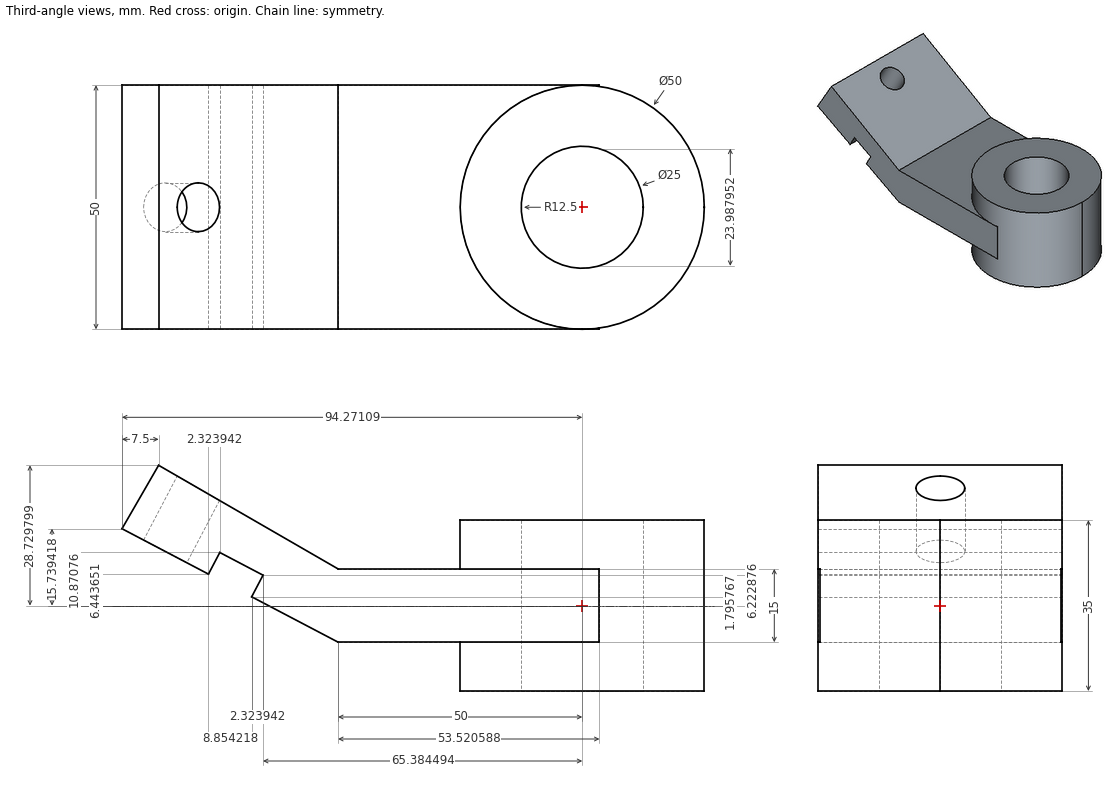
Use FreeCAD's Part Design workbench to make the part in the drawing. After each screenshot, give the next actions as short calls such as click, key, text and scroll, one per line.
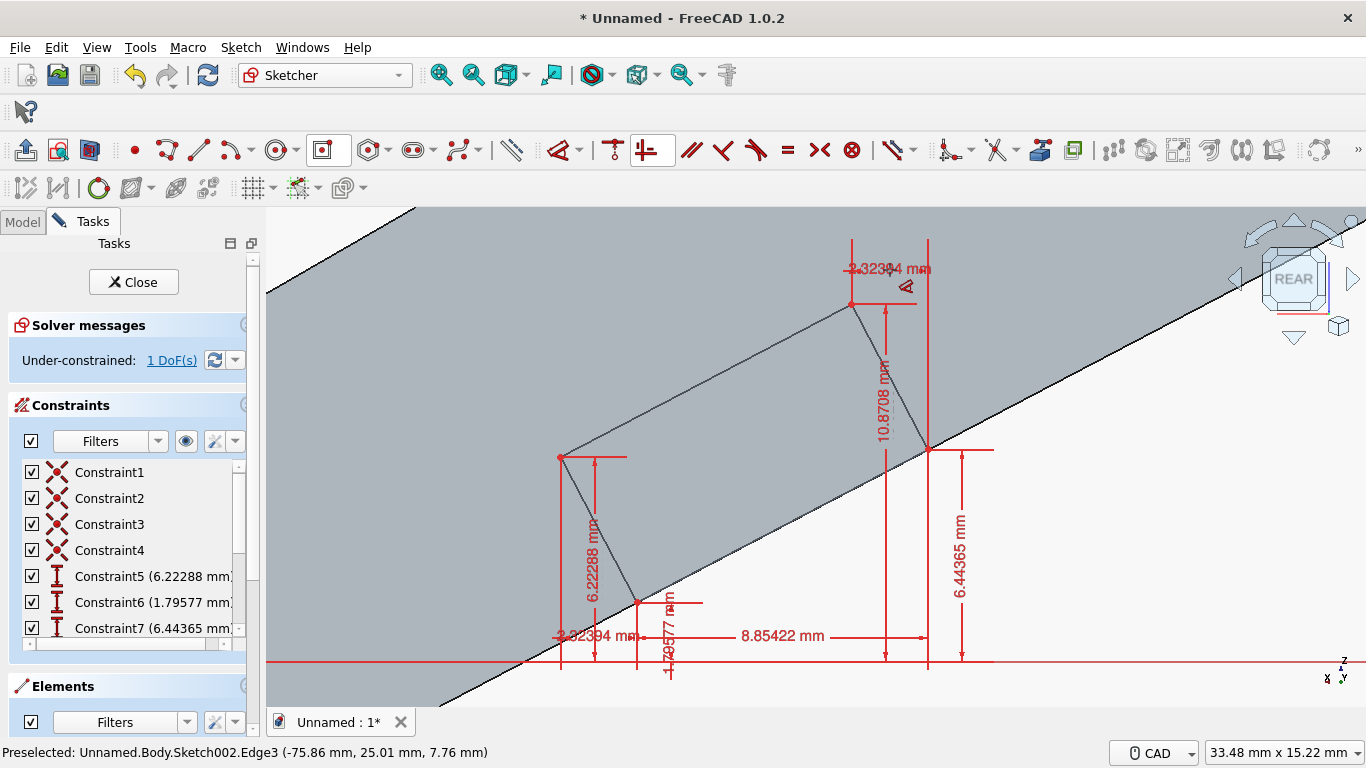
click(561, 457)
click(427, 423)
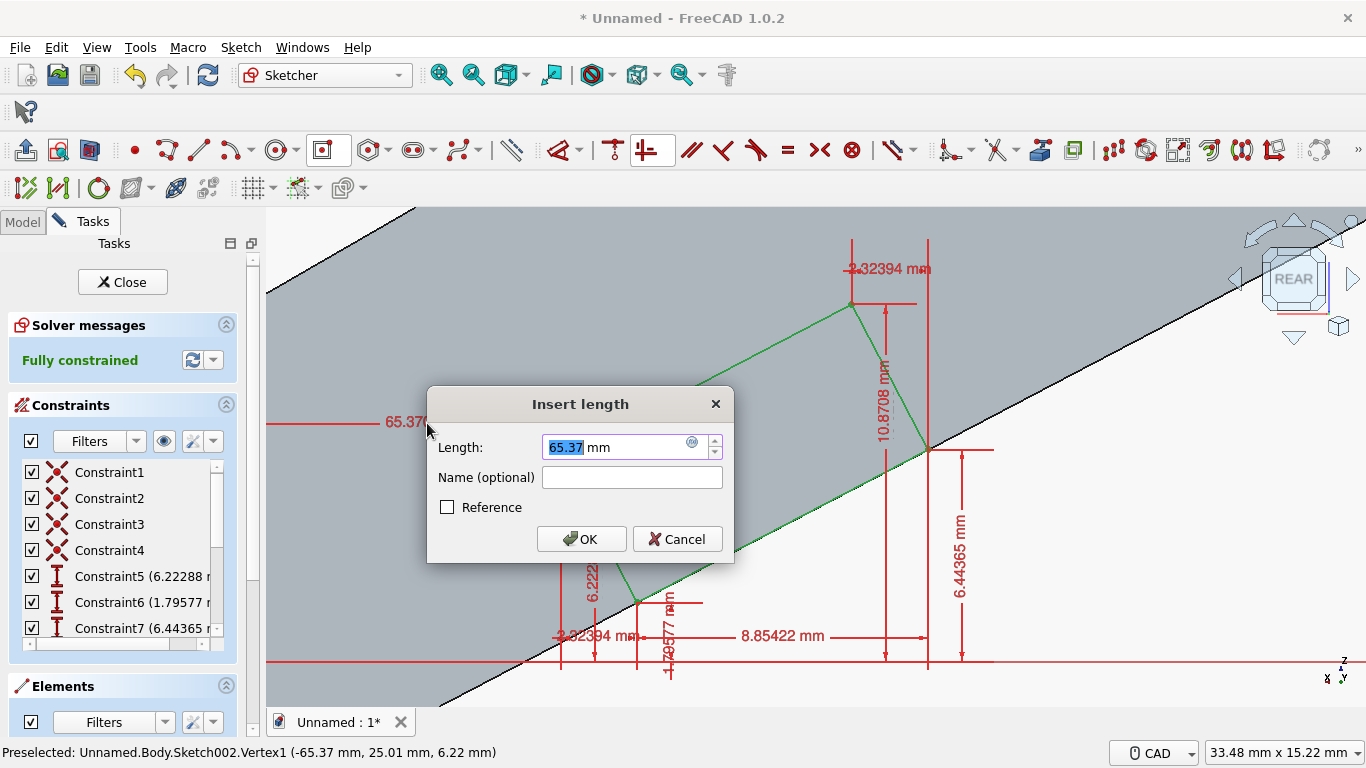
text(65.384494)
key(Return)
key(Escape)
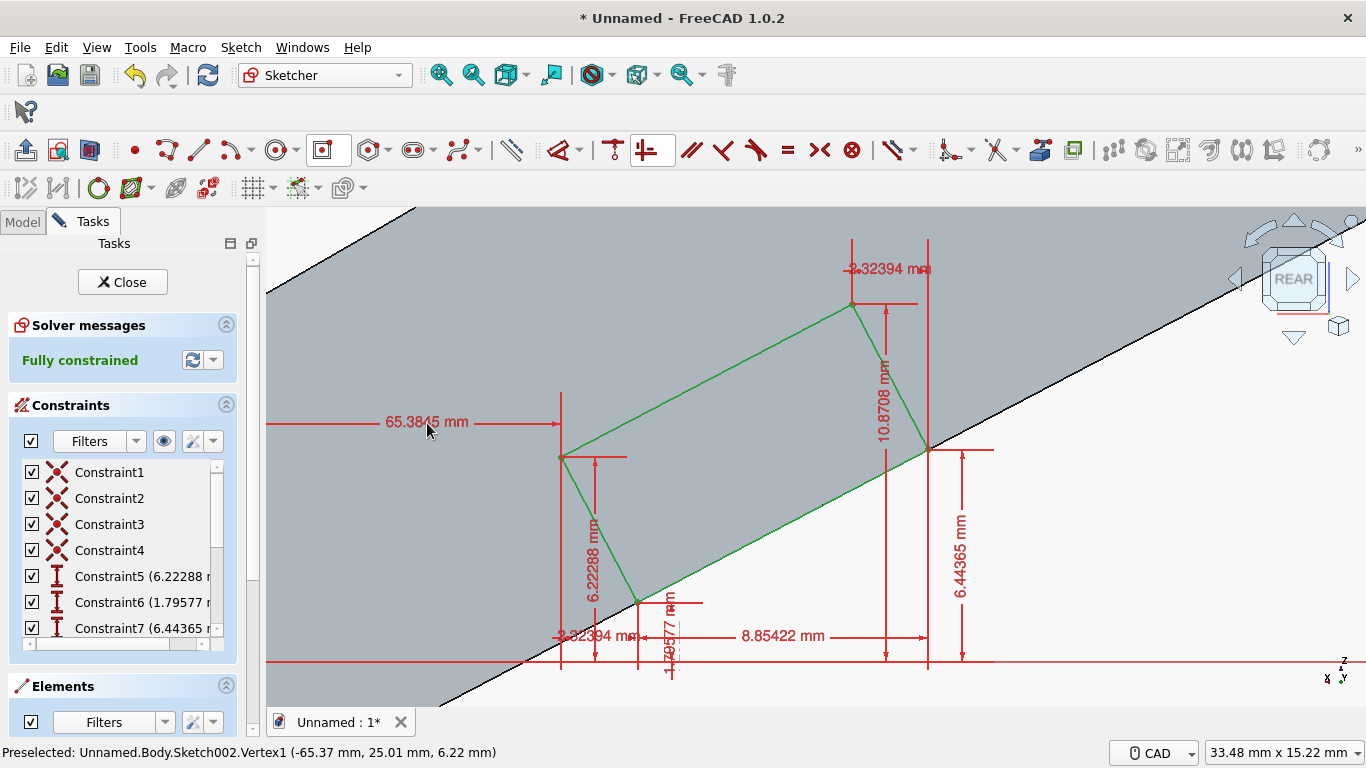
click(123, 282)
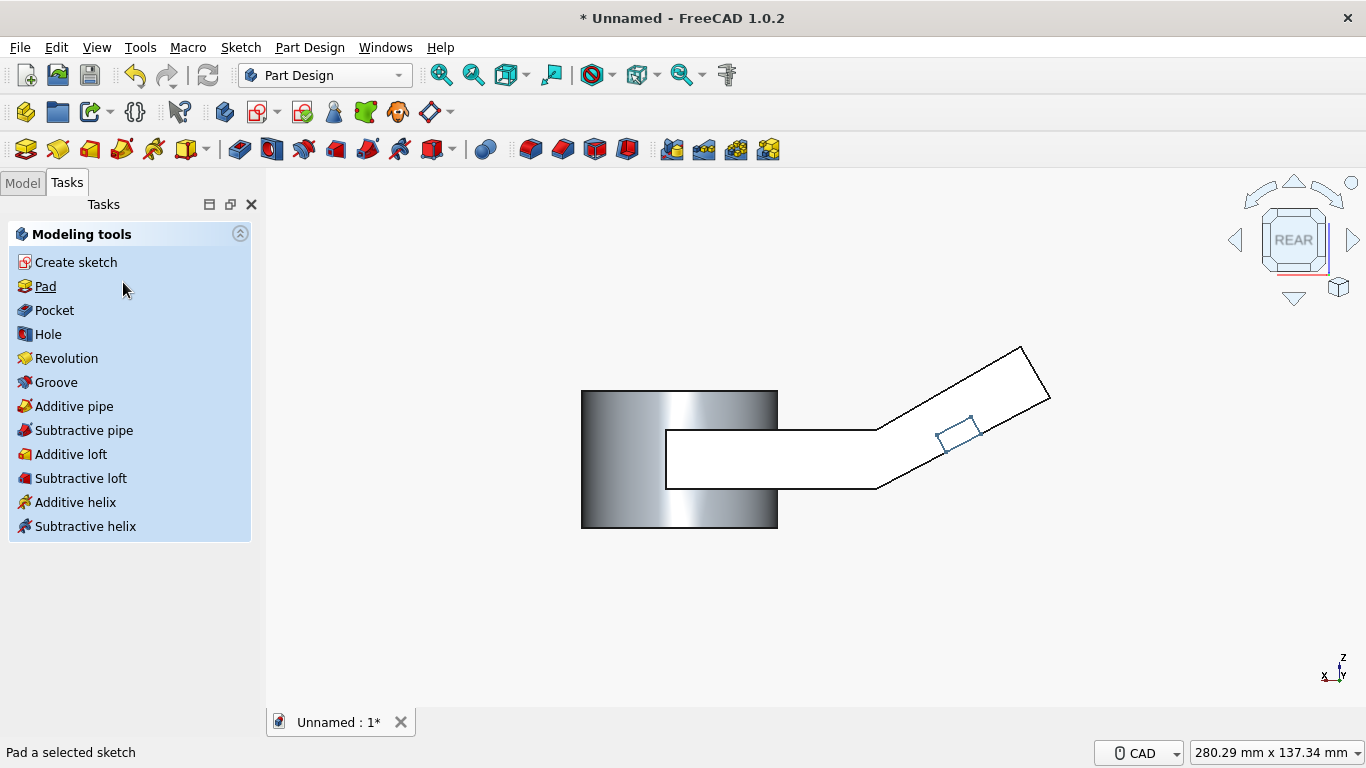
click(240, 150)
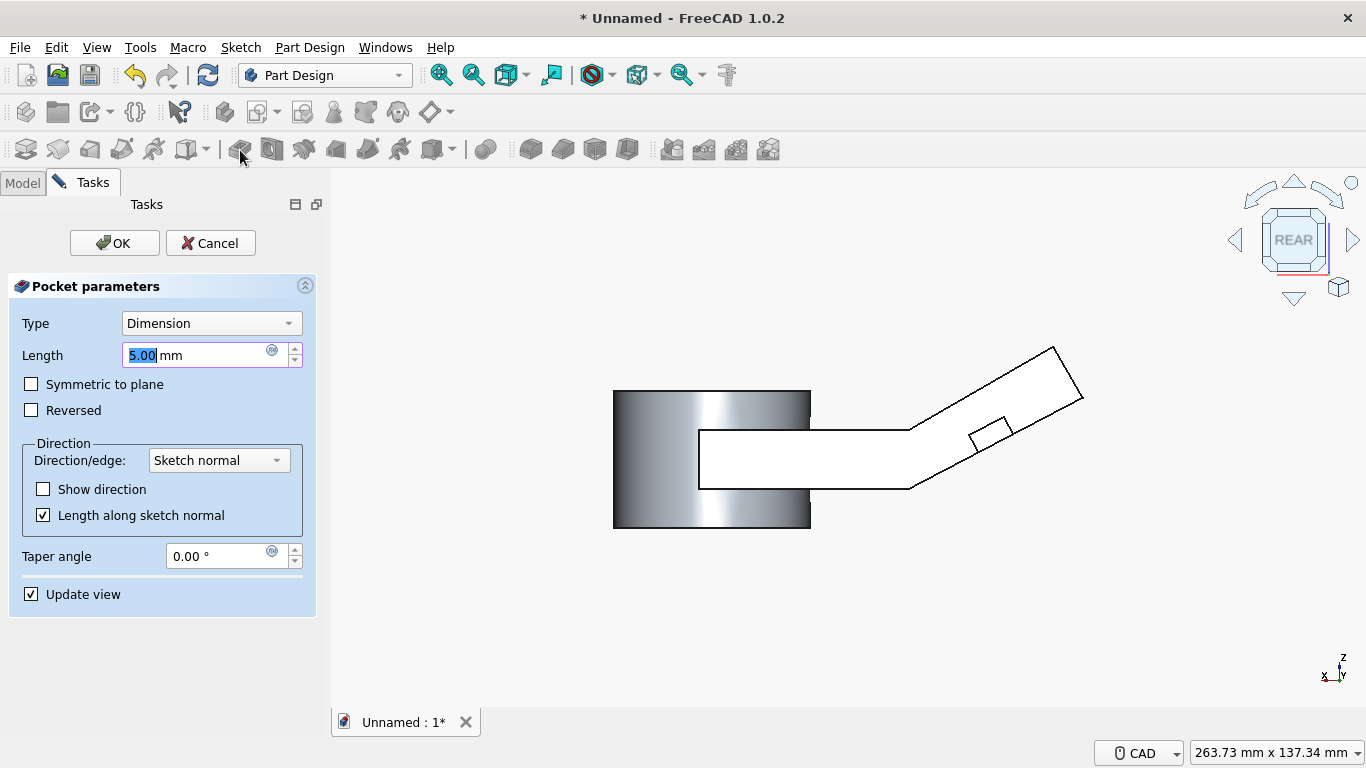
click(212, 324)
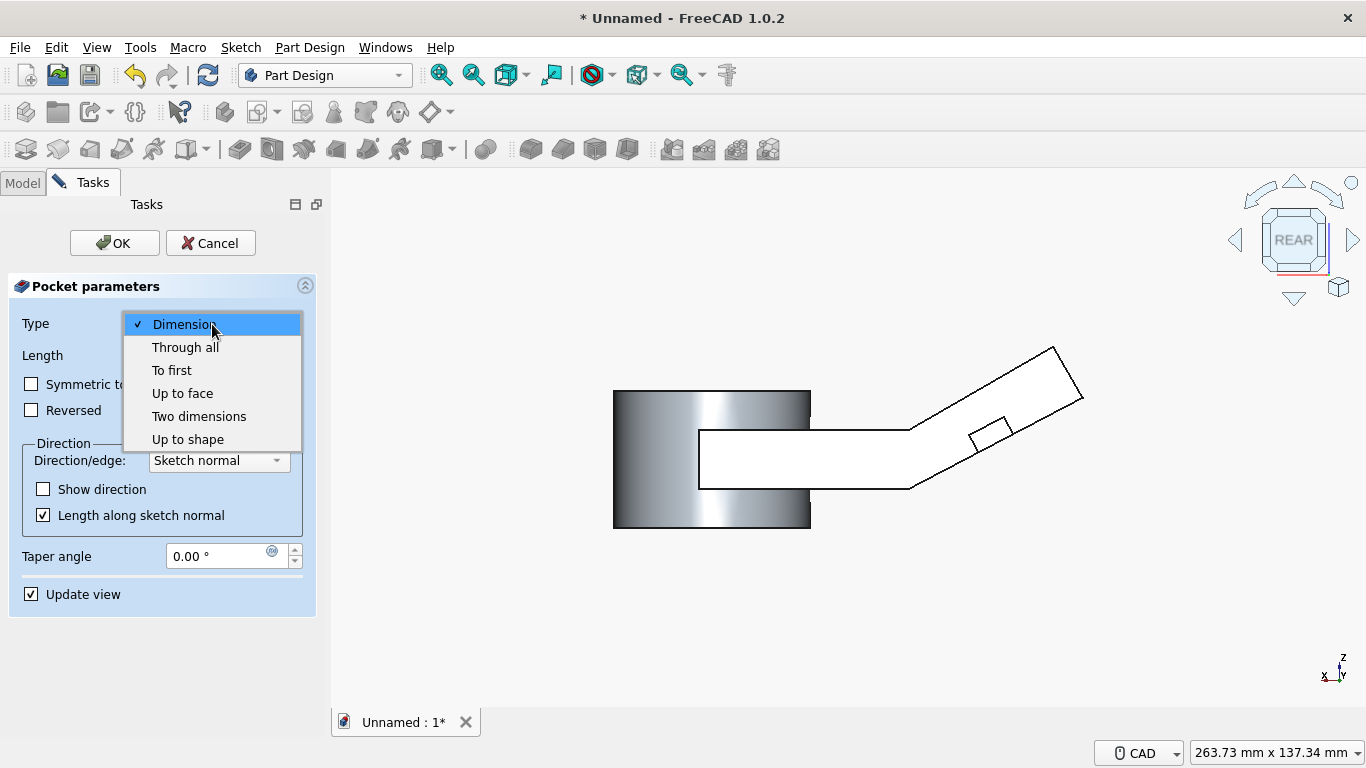
click(212, 348)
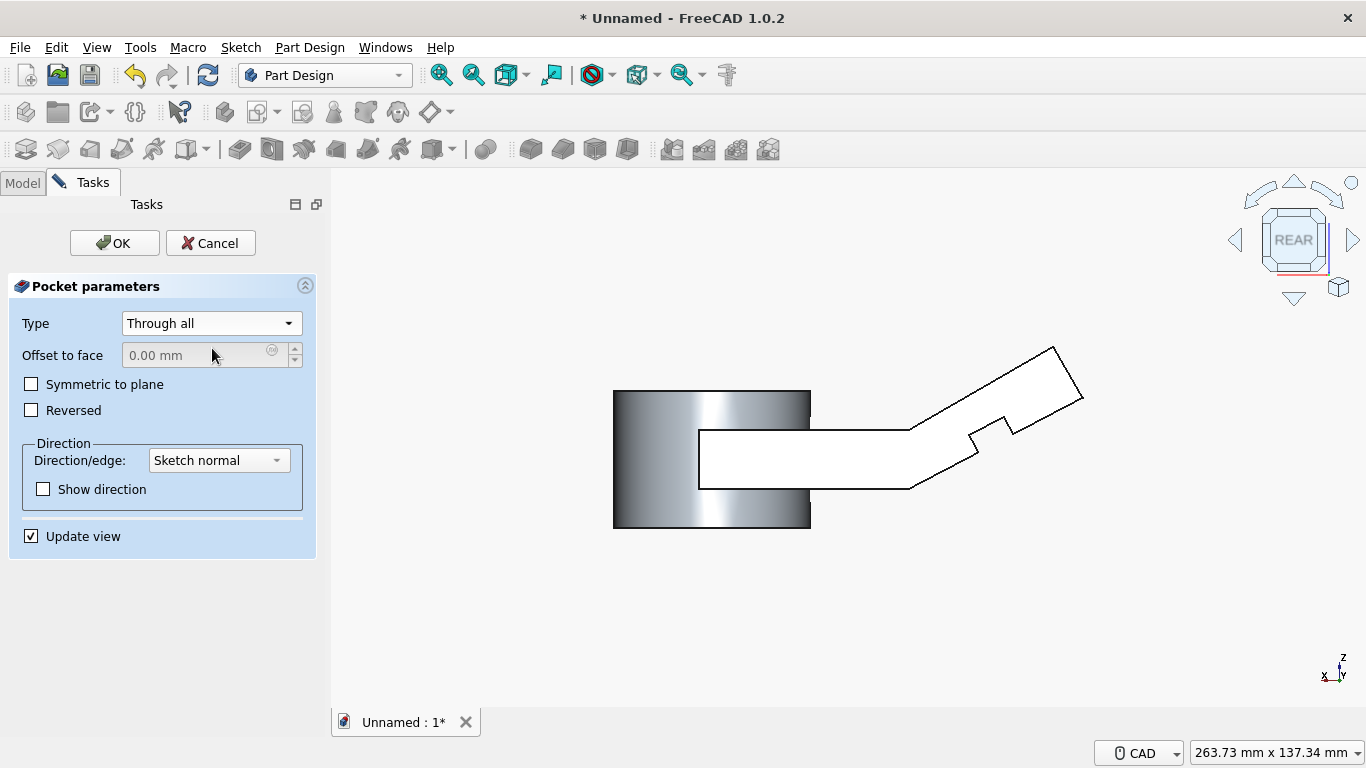
click(115, 243)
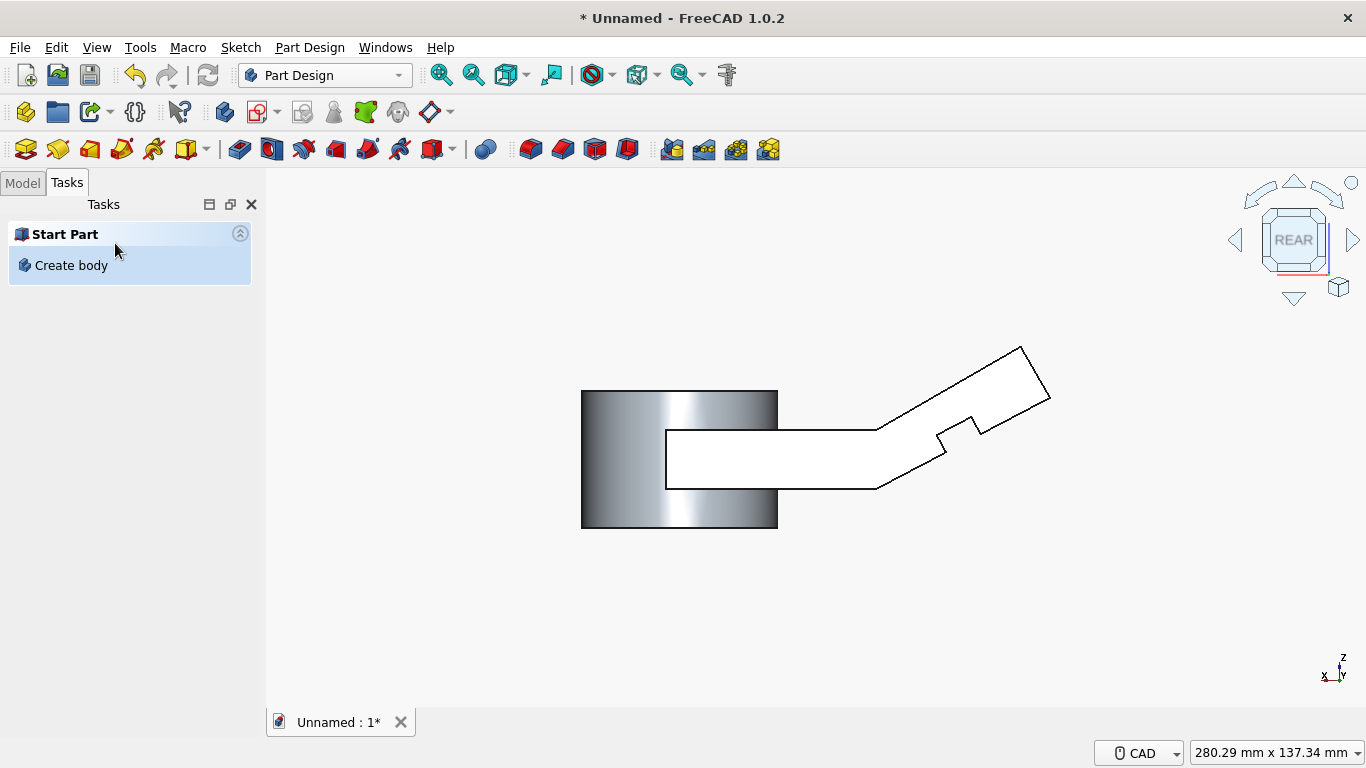
click(442, 76)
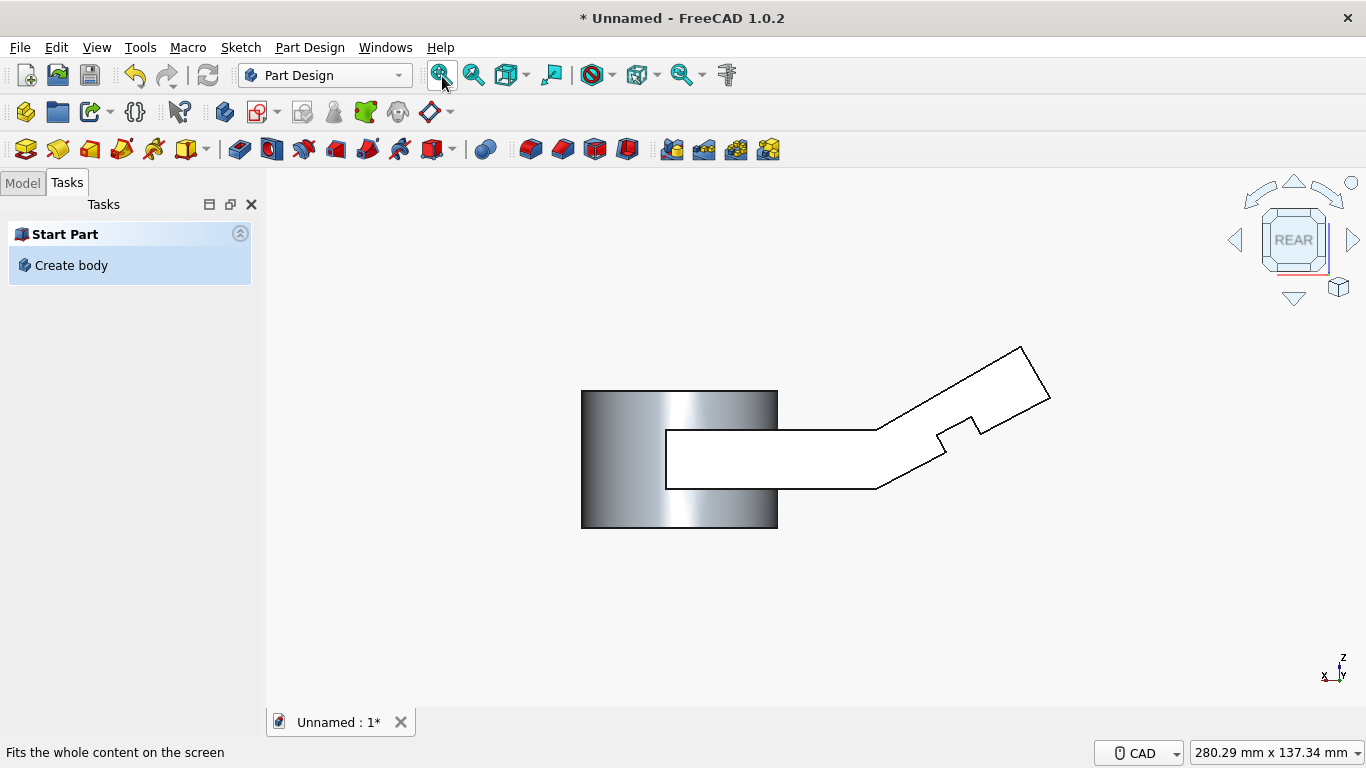
key(5)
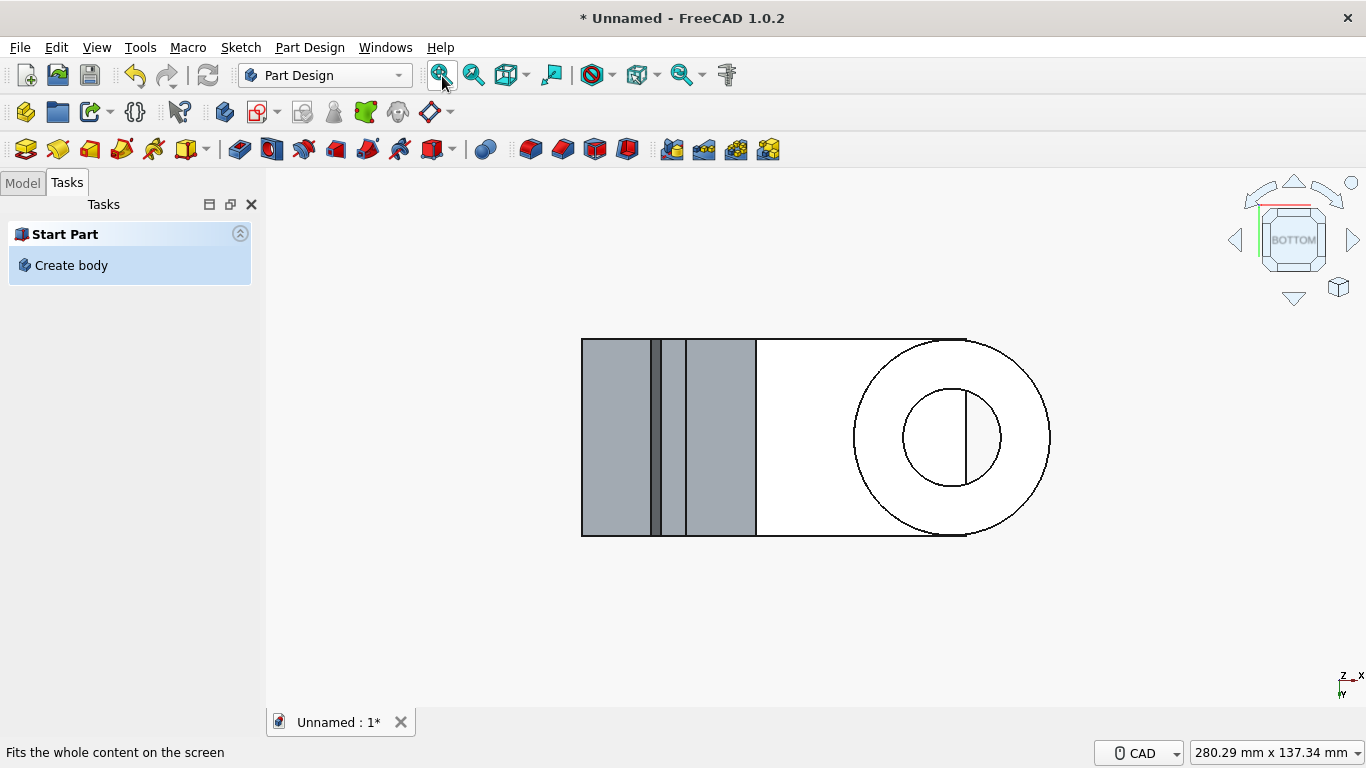
click(442, 76)